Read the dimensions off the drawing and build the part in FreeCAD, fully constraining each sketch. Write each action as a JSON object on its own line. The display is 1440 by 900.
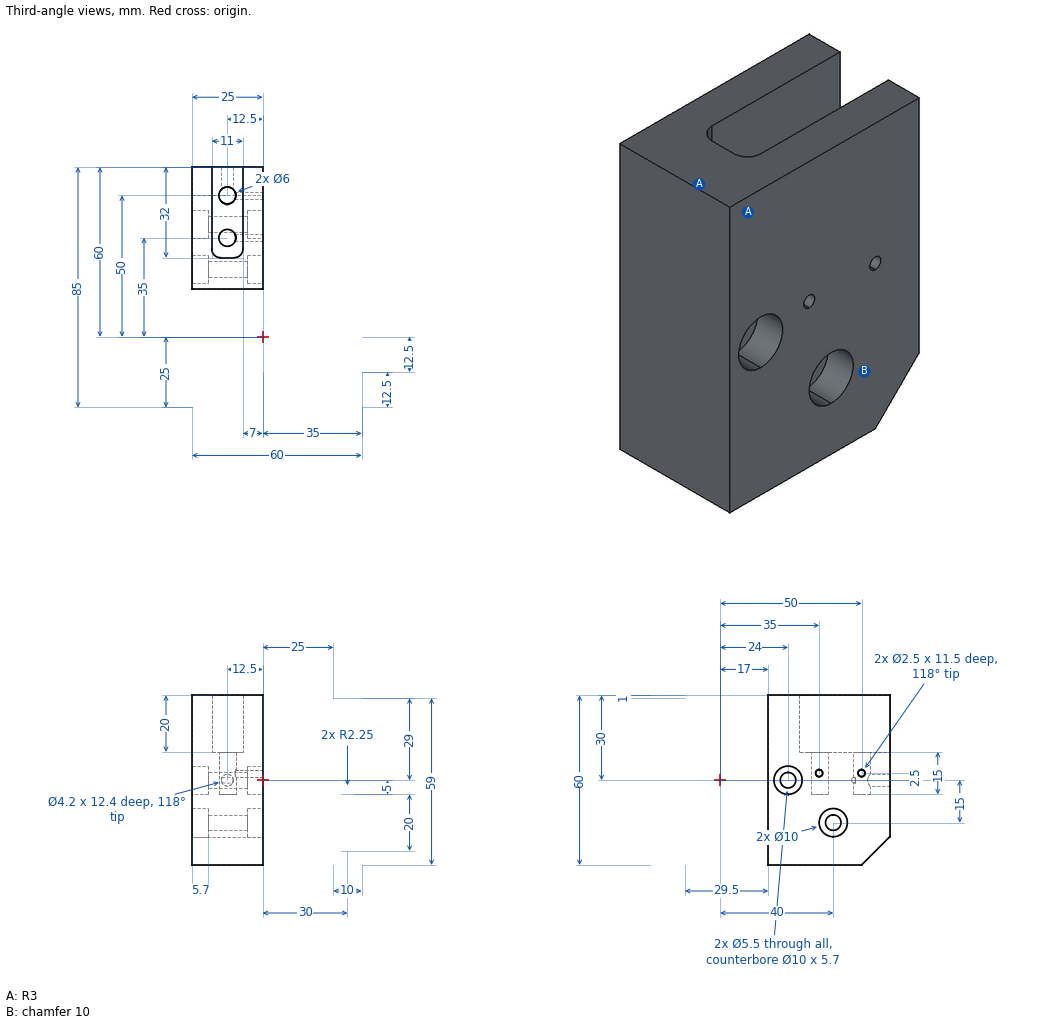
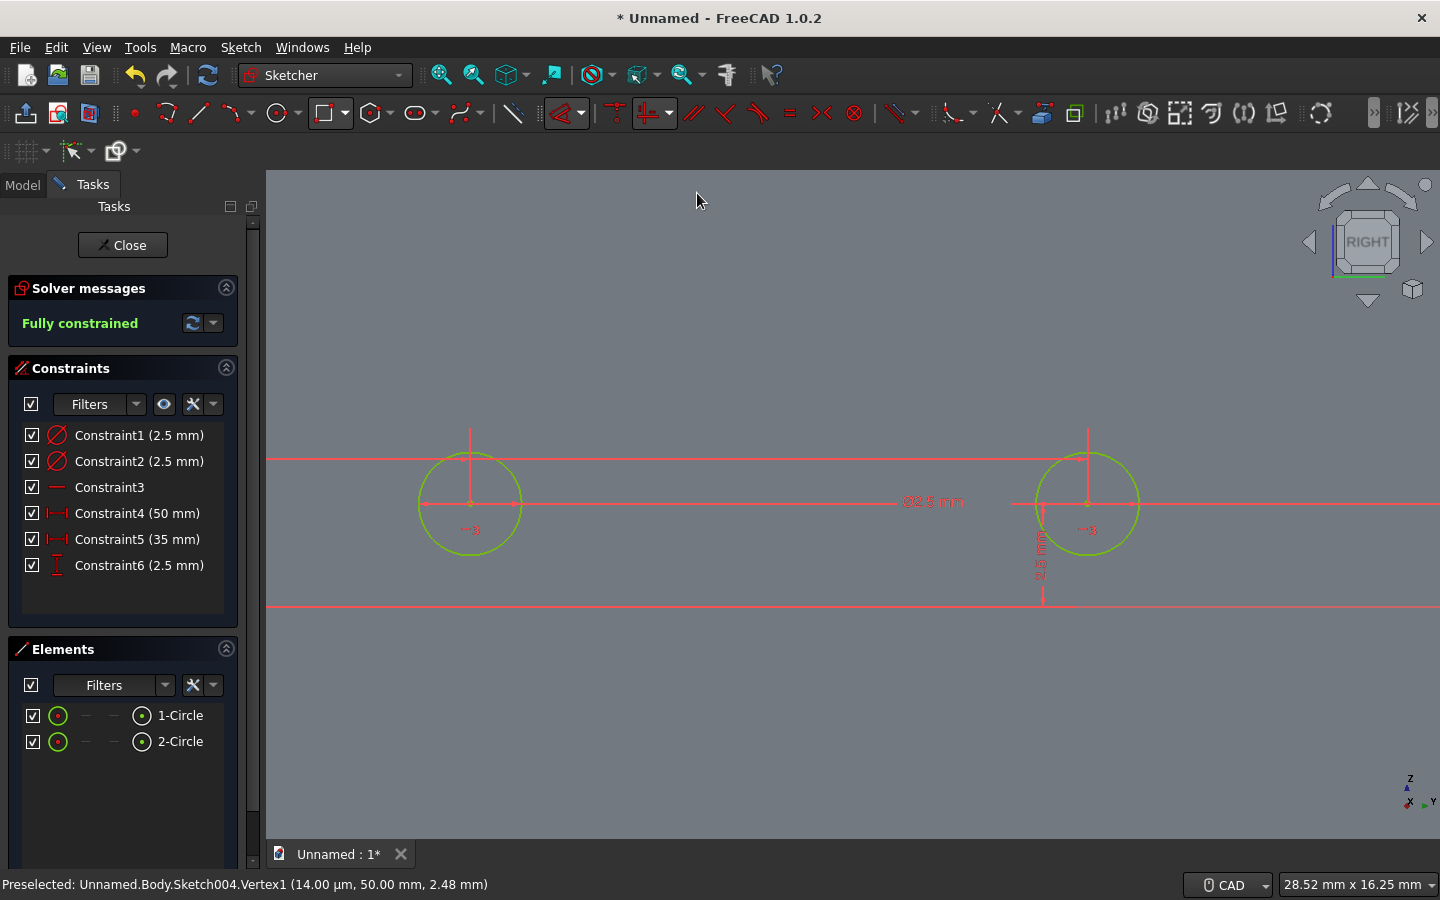
{"action": "left_click", "coordinate": [123, 245]}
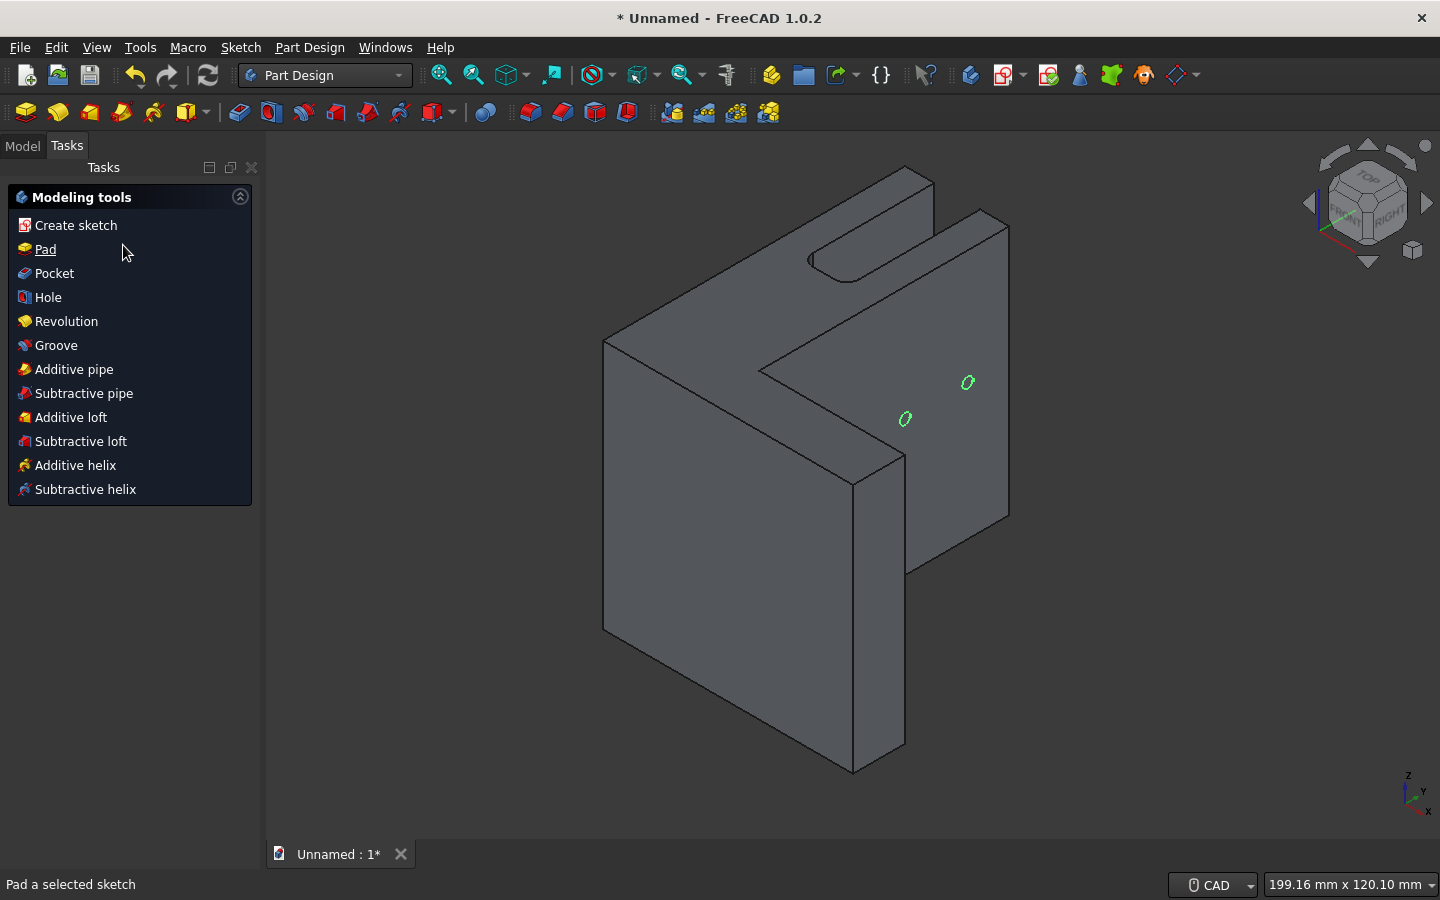
{"action": "left_click", "coordinate": [272, 112]}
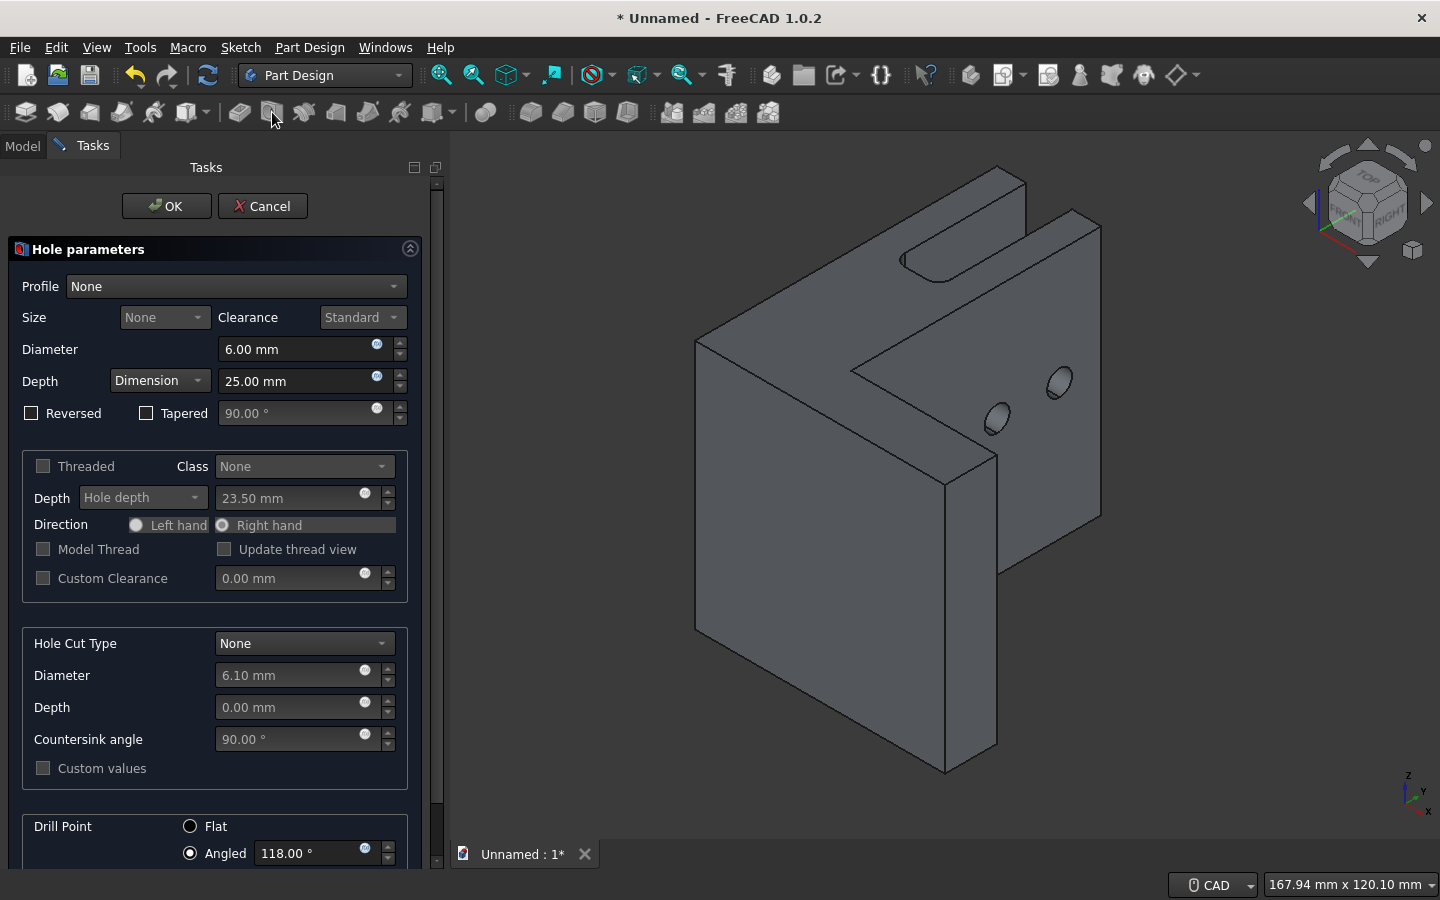
{"action": "triple_click", "coordinate": [305, 349]}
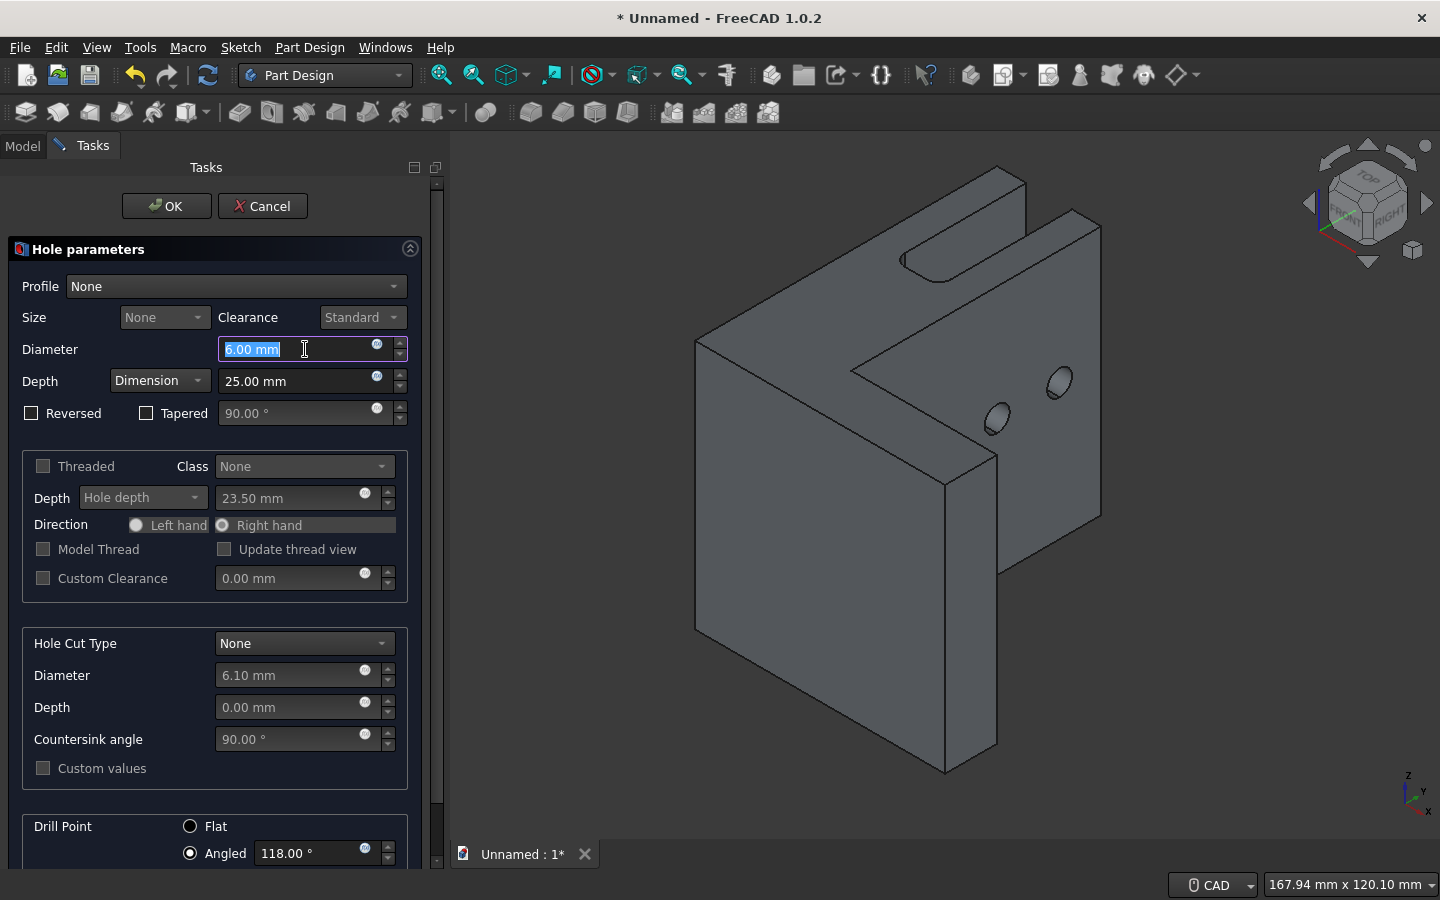
{"action": "type", "text": "2.5"}
{"action": "key", "text": "Tab"}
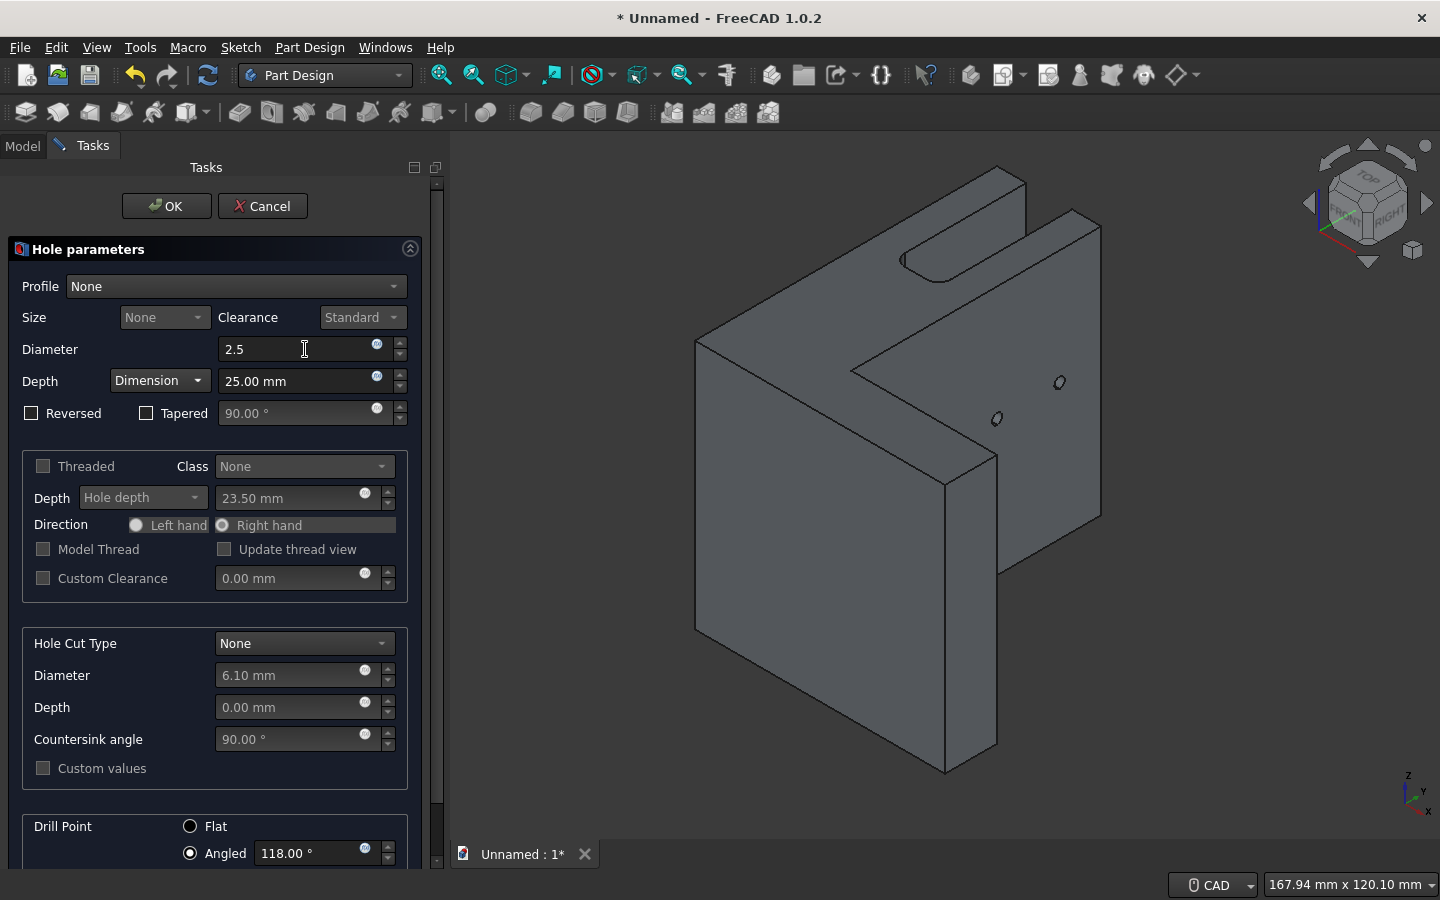
{"action": "triple_click", "coordinate": [305, 381]}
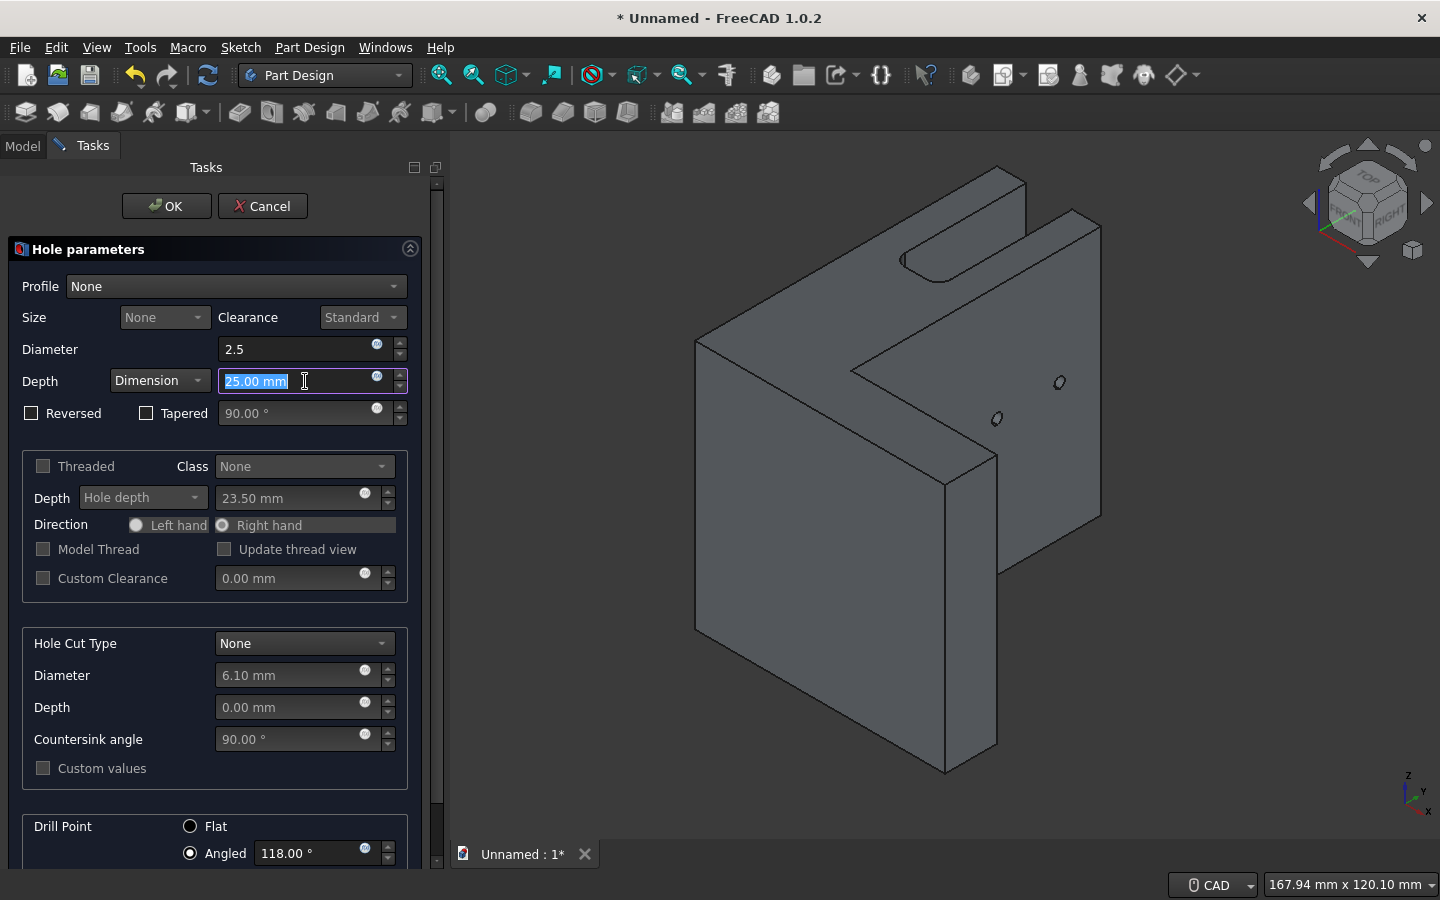
{"action": "type", "text": "11.5"}
{"action": "key", "text": "Tab"}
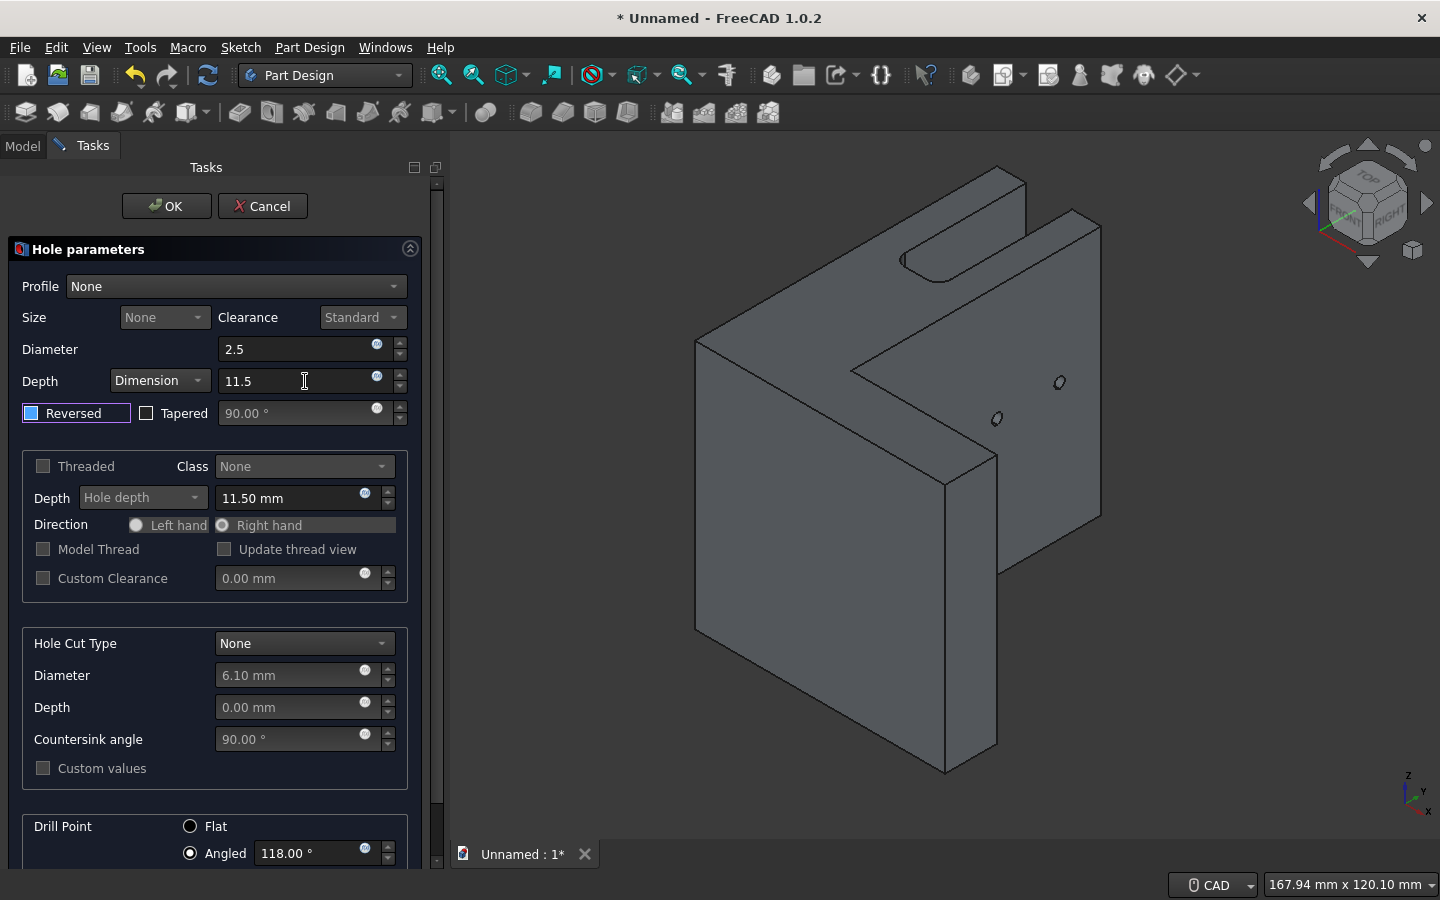
{"action": "left_click", "coordinate": [167, 206]}